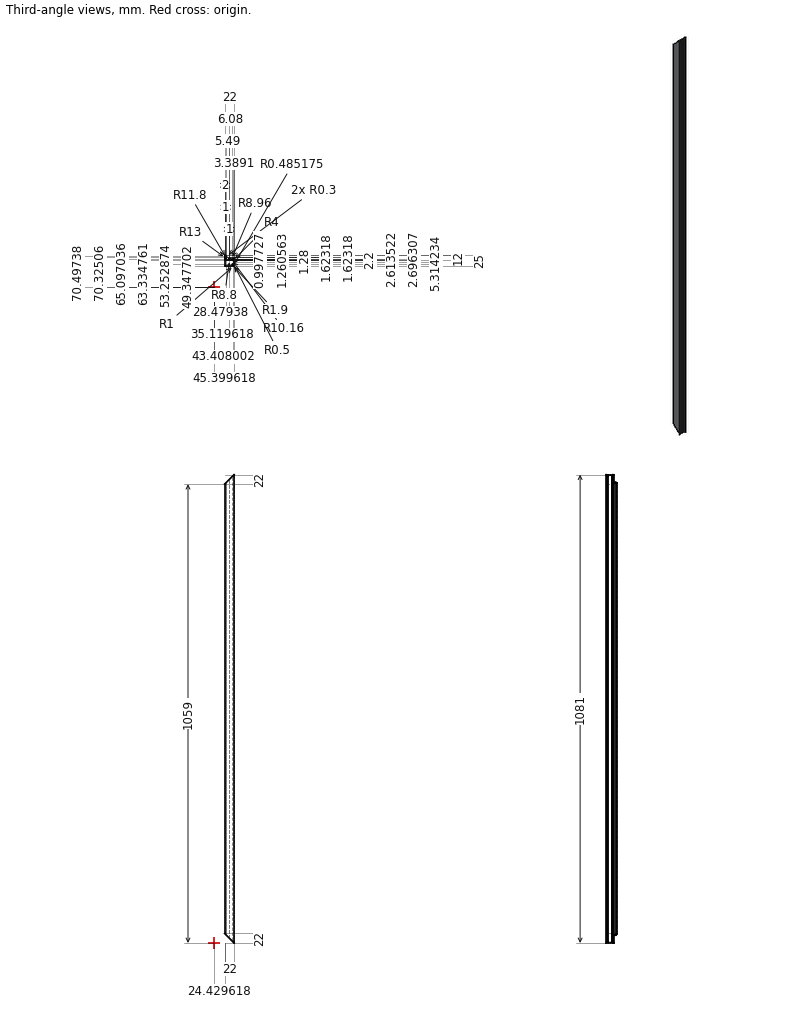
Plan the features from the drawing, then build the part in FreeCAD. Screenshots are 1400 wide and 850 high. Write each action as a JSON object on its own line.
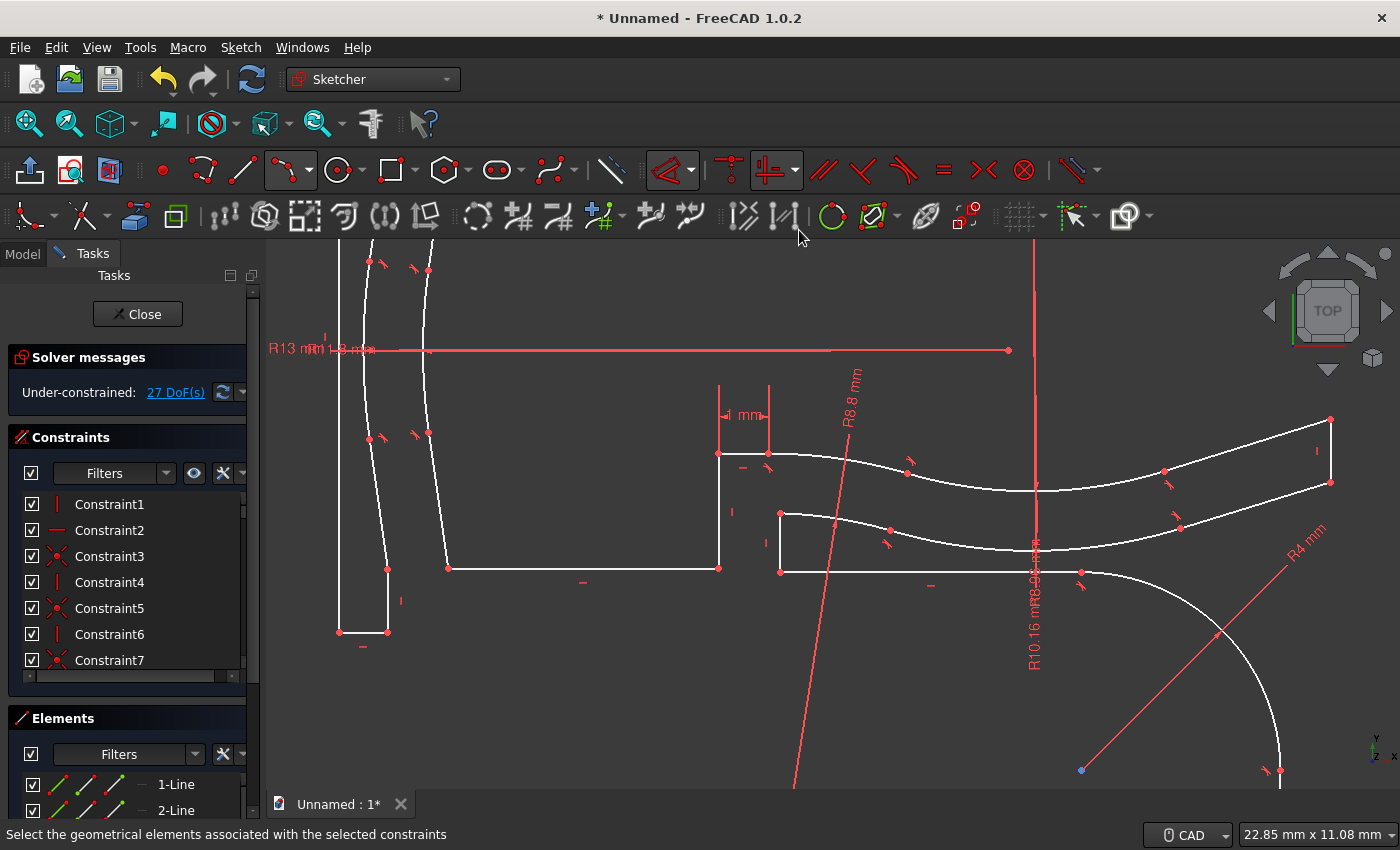
{"action": "left_click", "coordinate": [373, 633]}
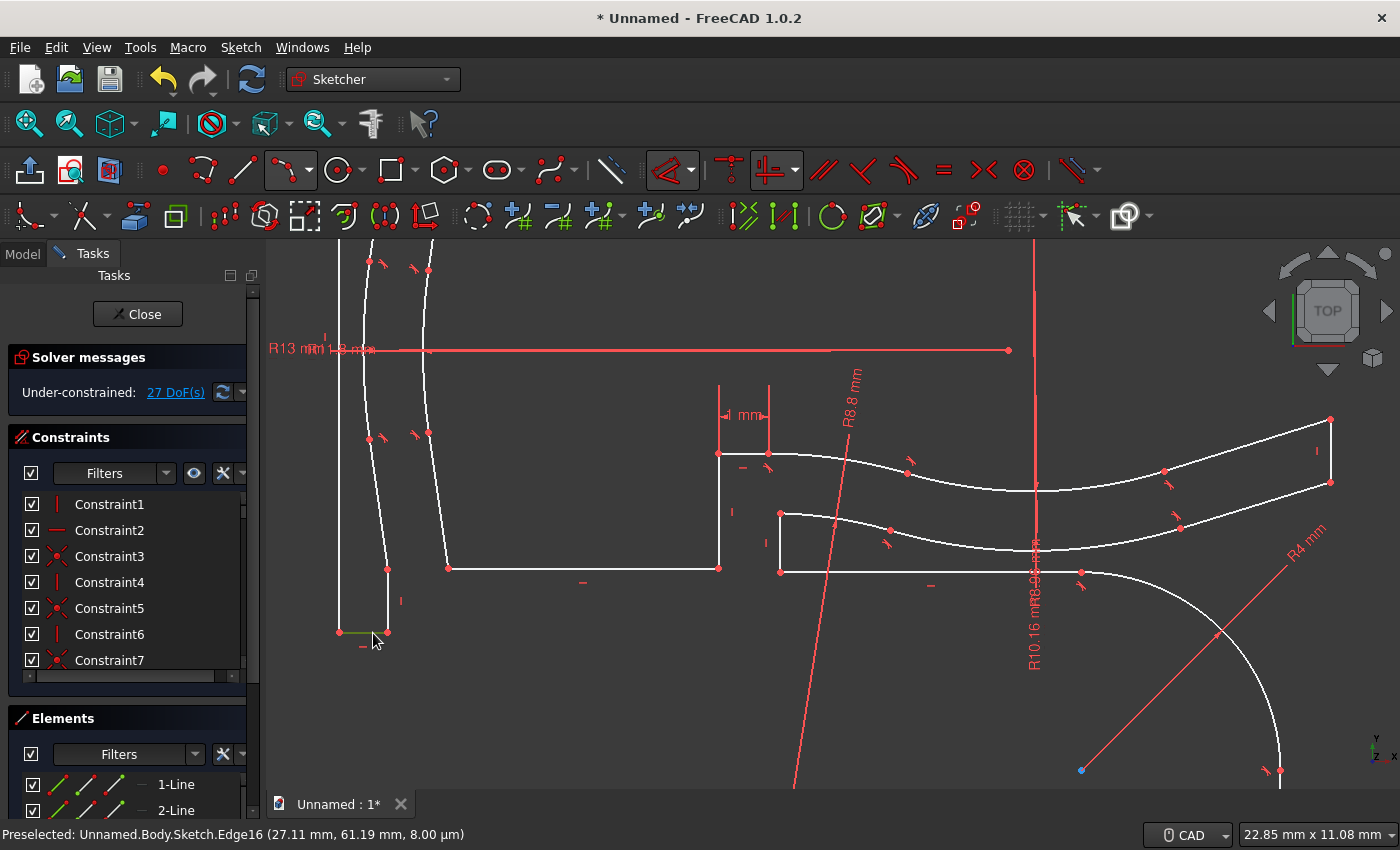
{"action": "key", "text": "l"}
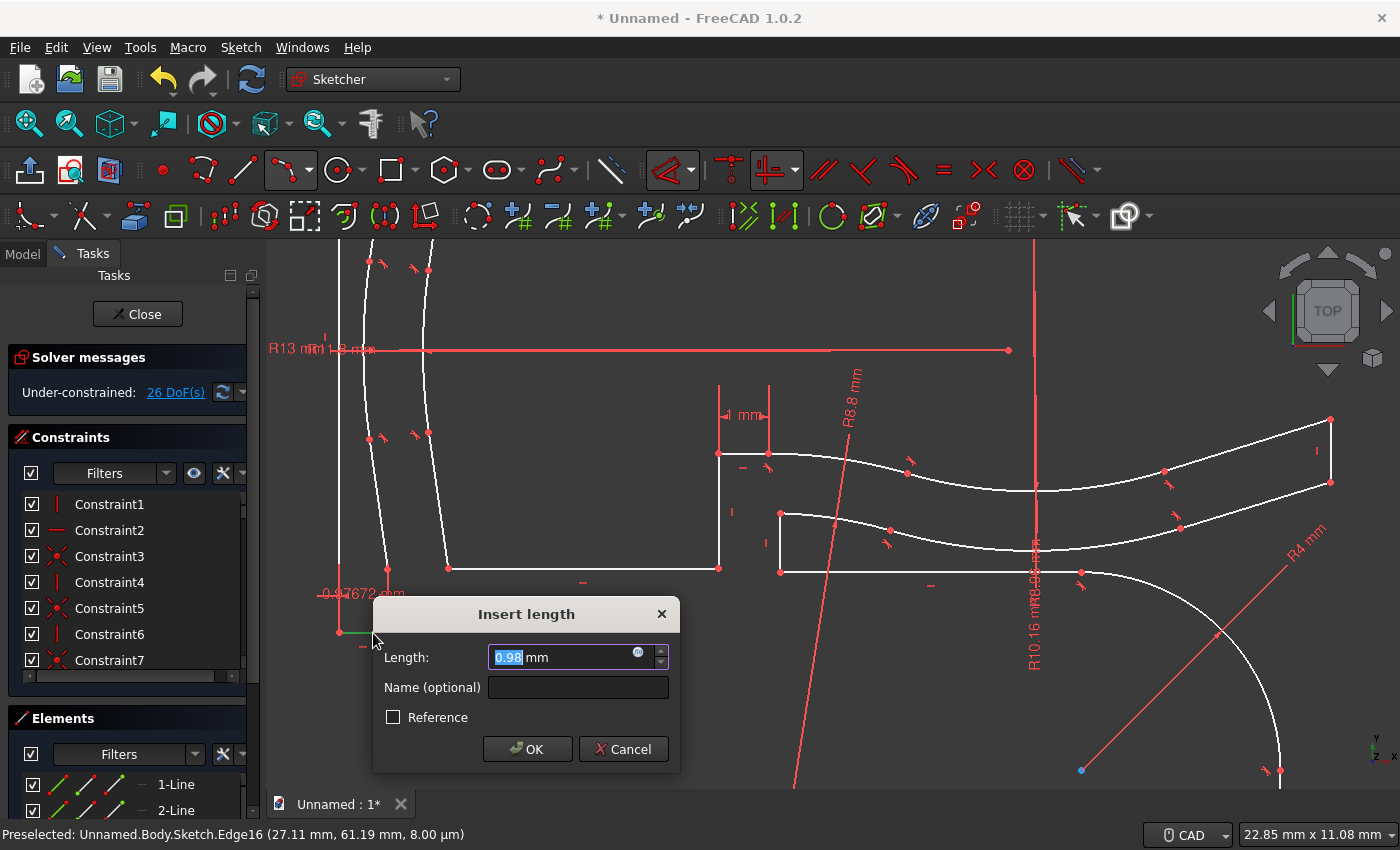
{"action": "type", "text": "1"}
{"action": "key", "text": "Return"}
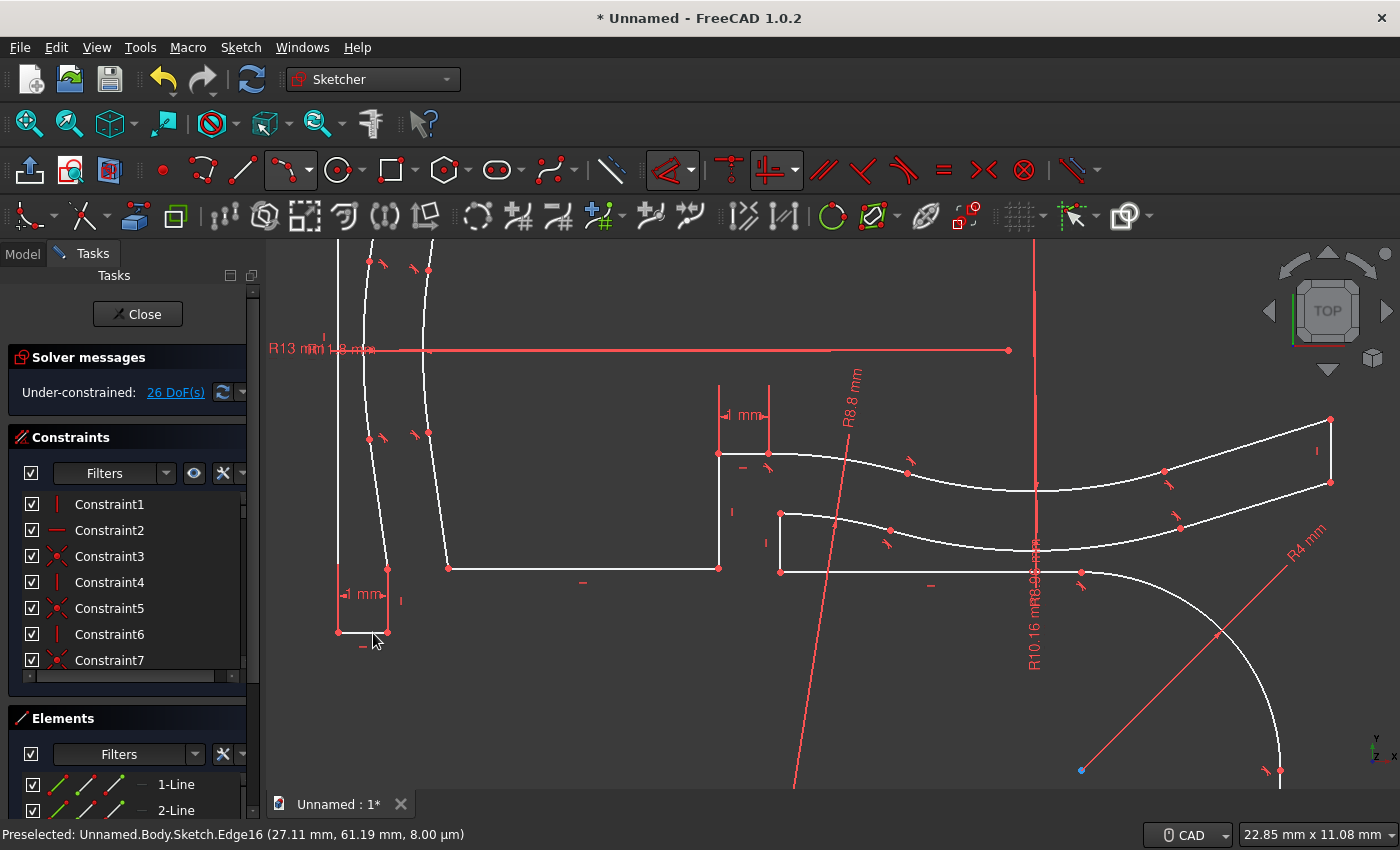
{"action": "scroll", "coordinate": [755, 452], "scroll_direction": "down", "scroll_amount": 6}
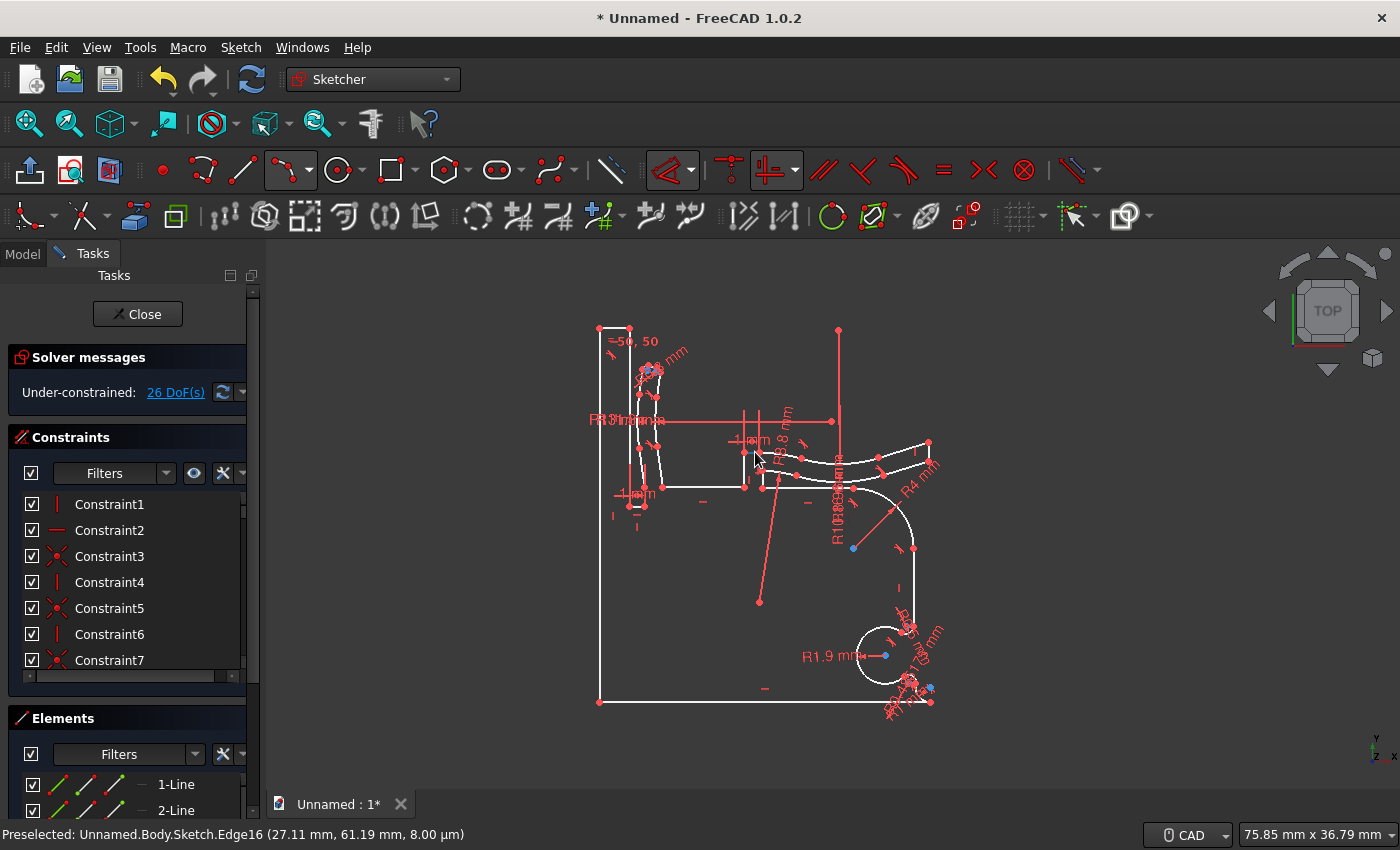
{"action": "scroll", "coordinate": [621, 328], "scroll_direction": "up", "scroll_amount": 3}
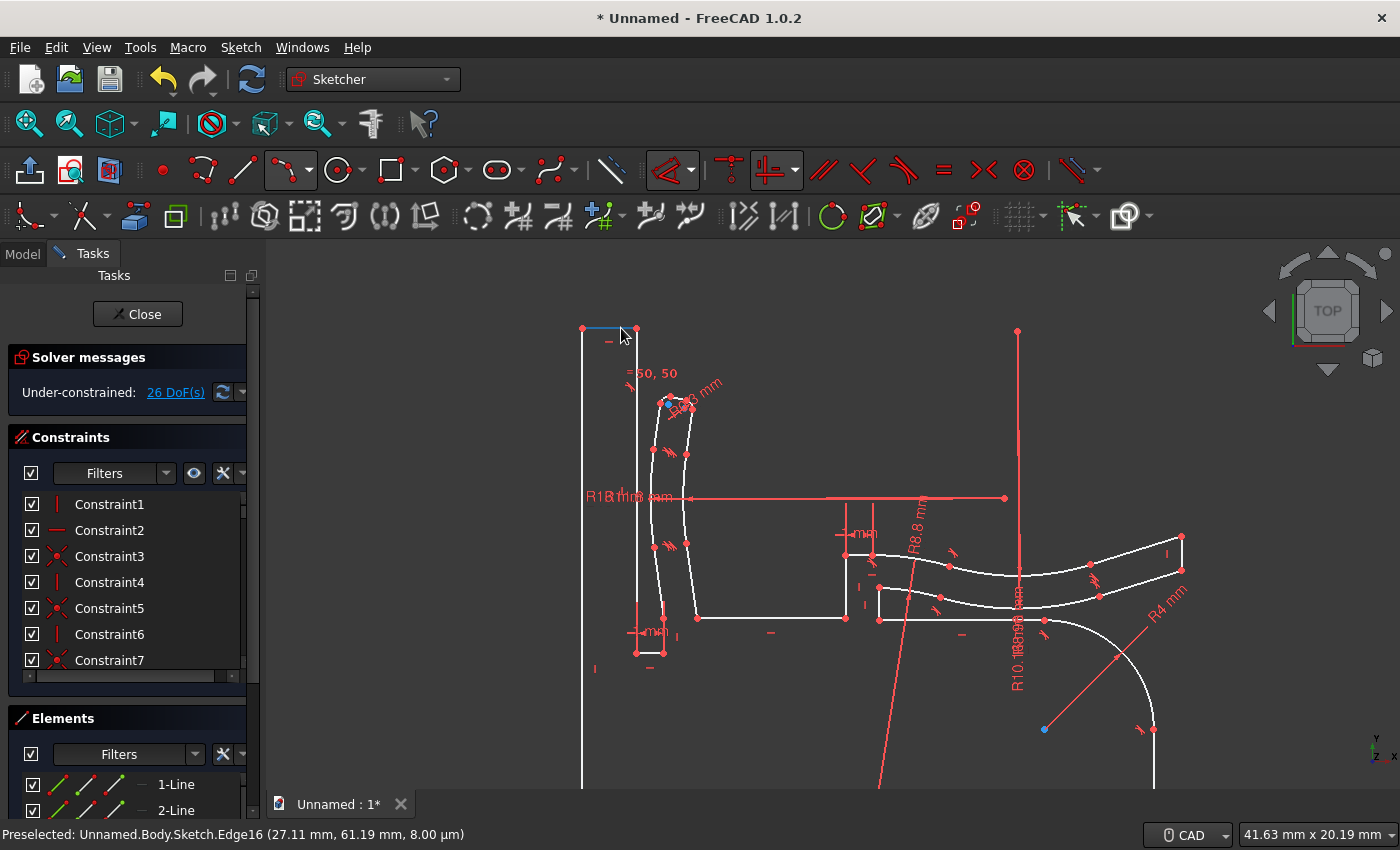
{"action": "left_click", "coordinate": [620, 328]}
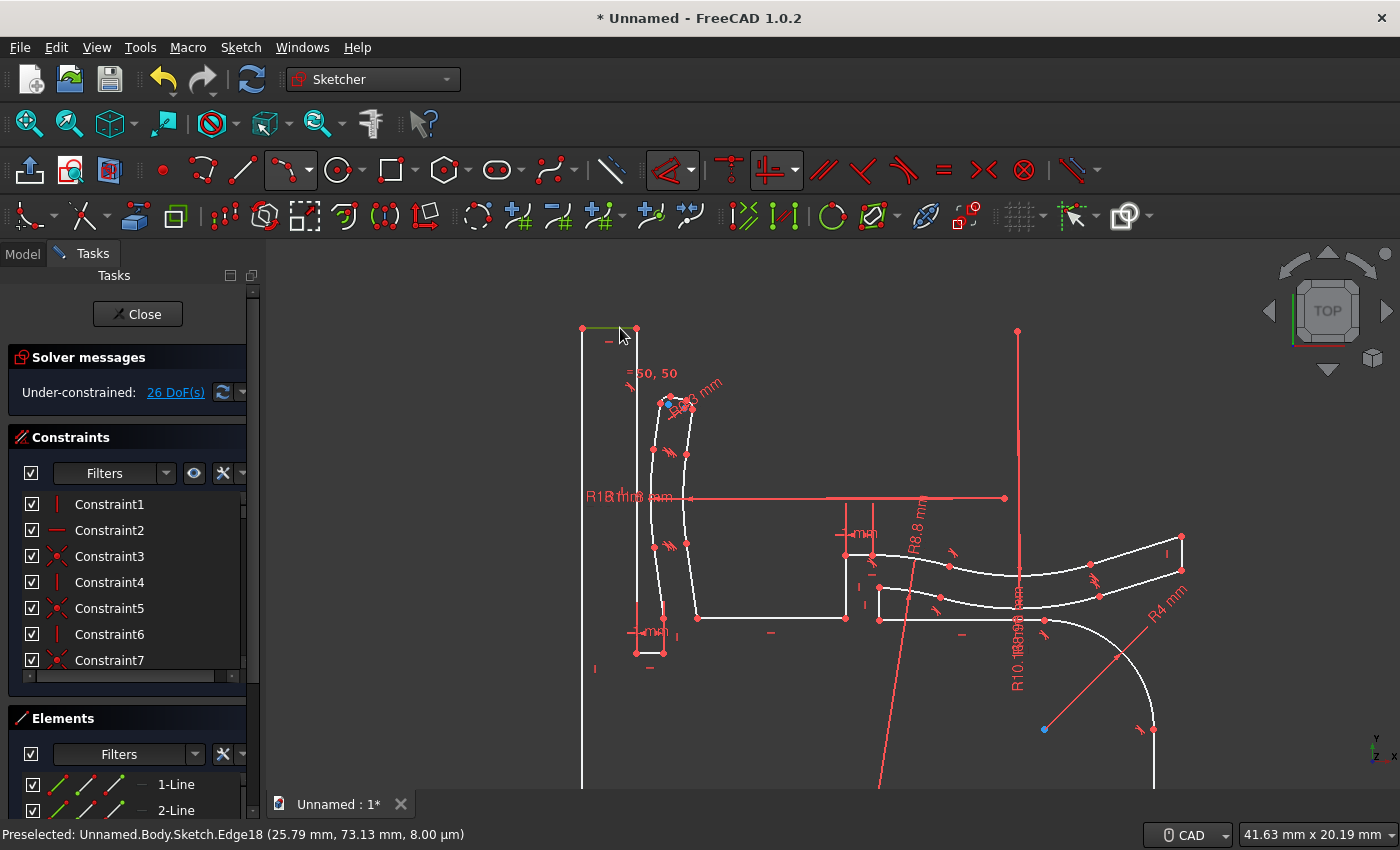
{"action": "key", "text": "l"}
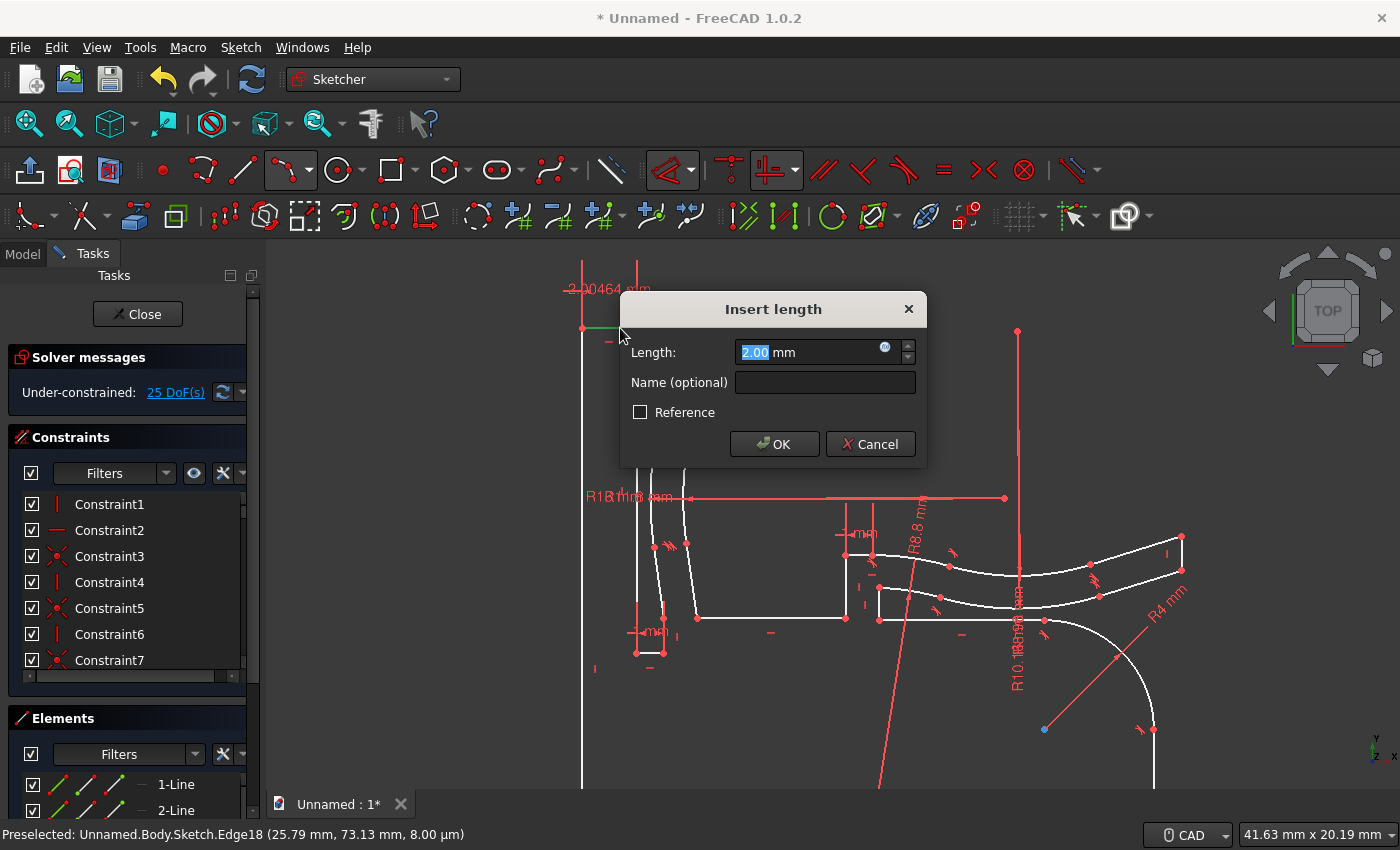
{"action": "type", "text": "2"}
{"action": "key", "text": "Return"}